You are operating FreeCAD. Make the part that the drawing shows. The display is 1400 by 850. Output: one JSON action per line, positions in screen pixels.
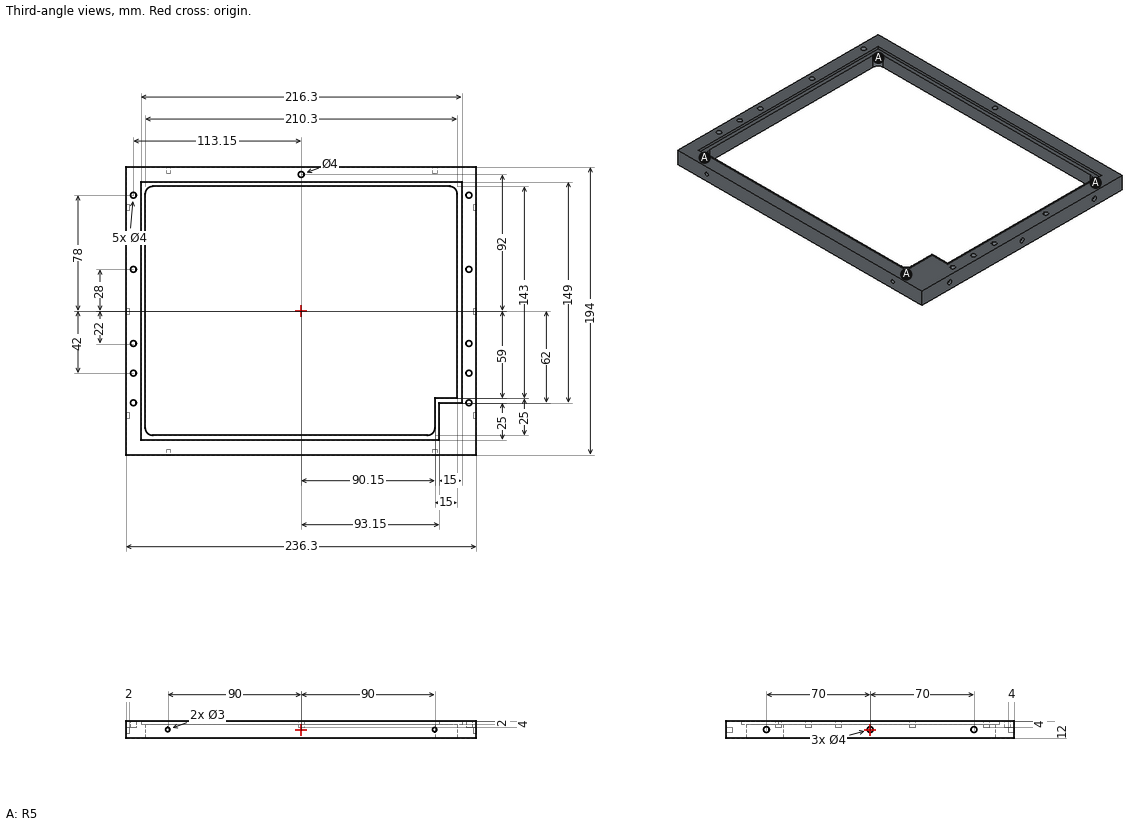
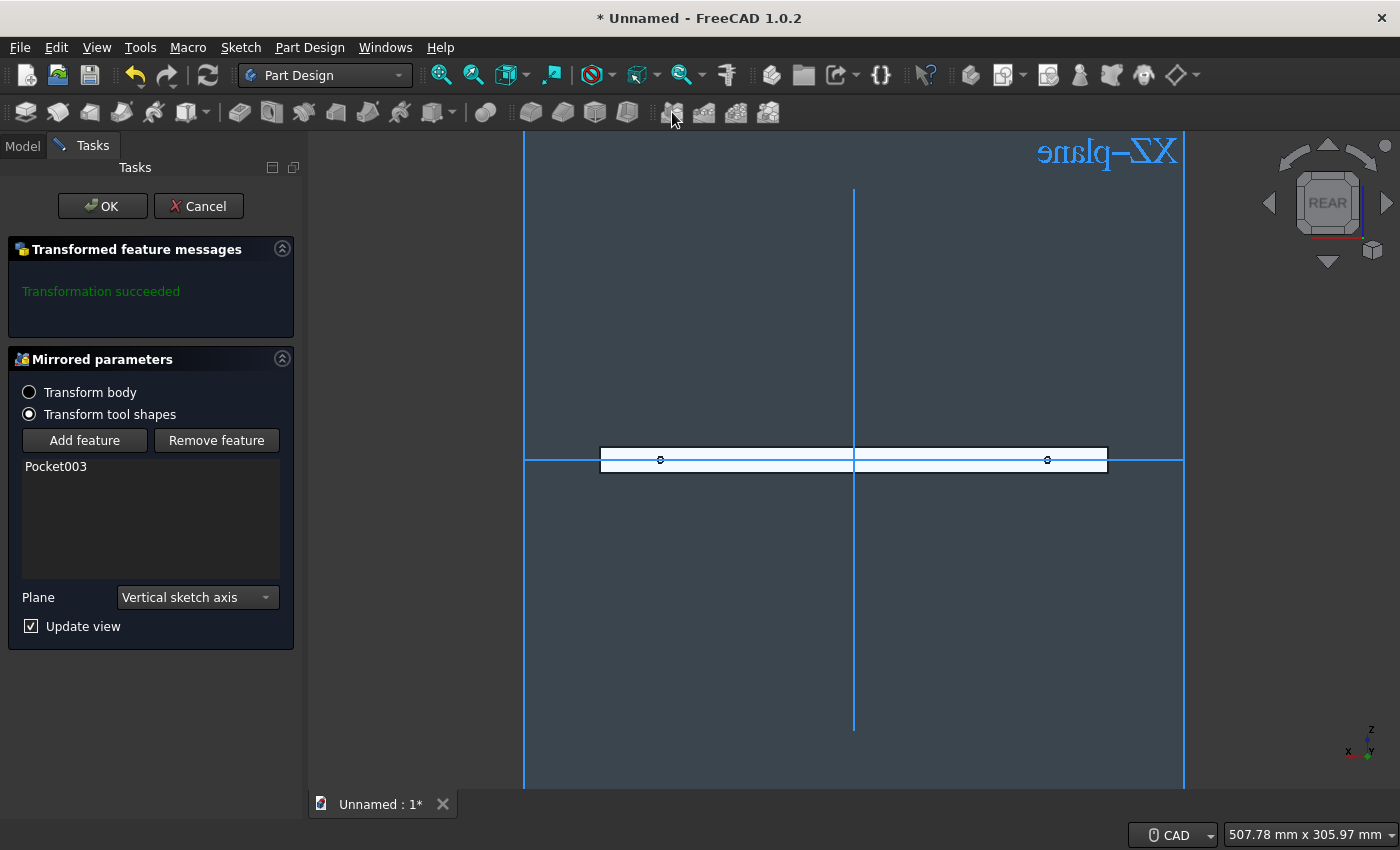
{"action": "left_click", "coordinate": [198, 598]}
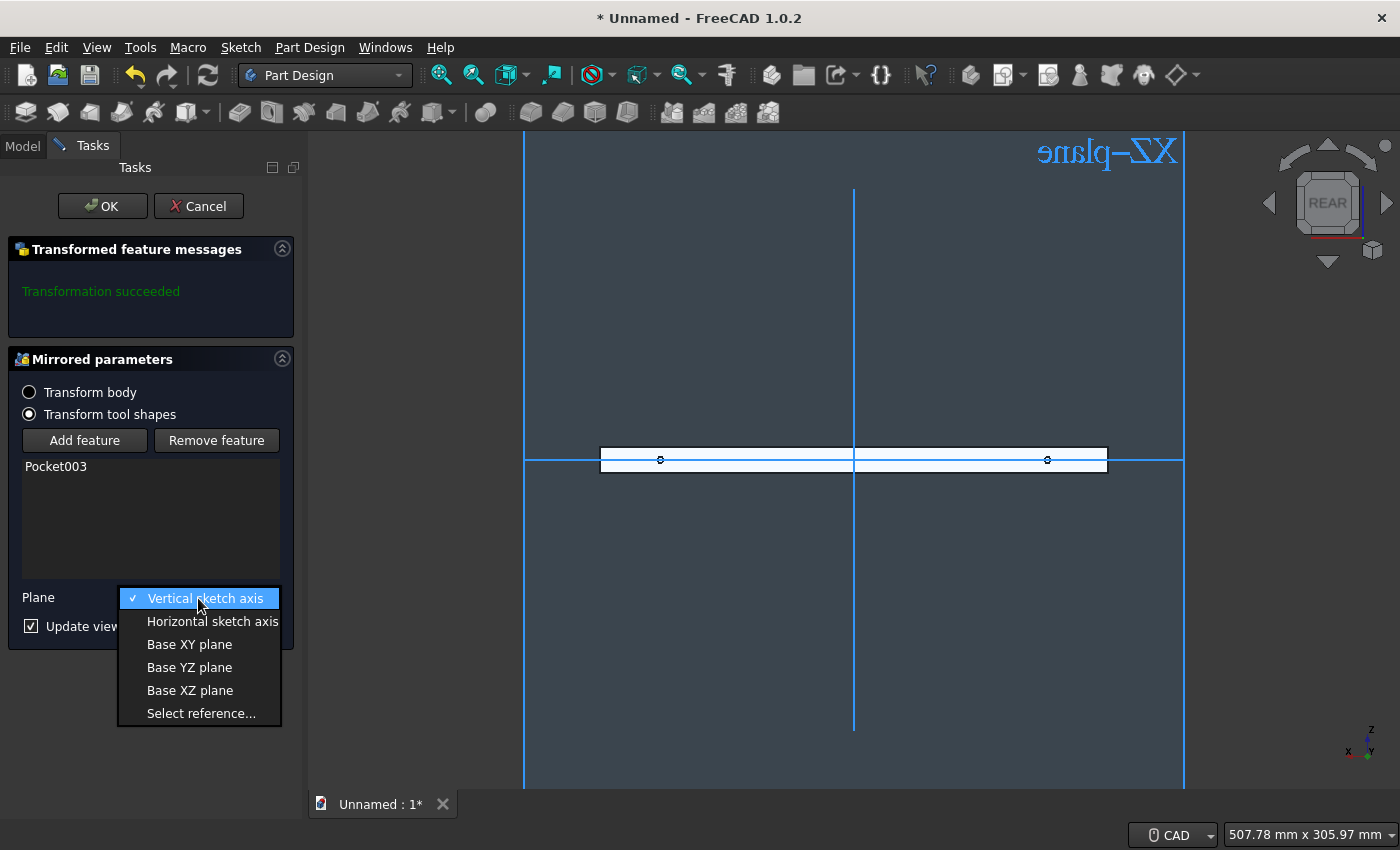
{"action": "left_click", "coordinate": [198, 690]}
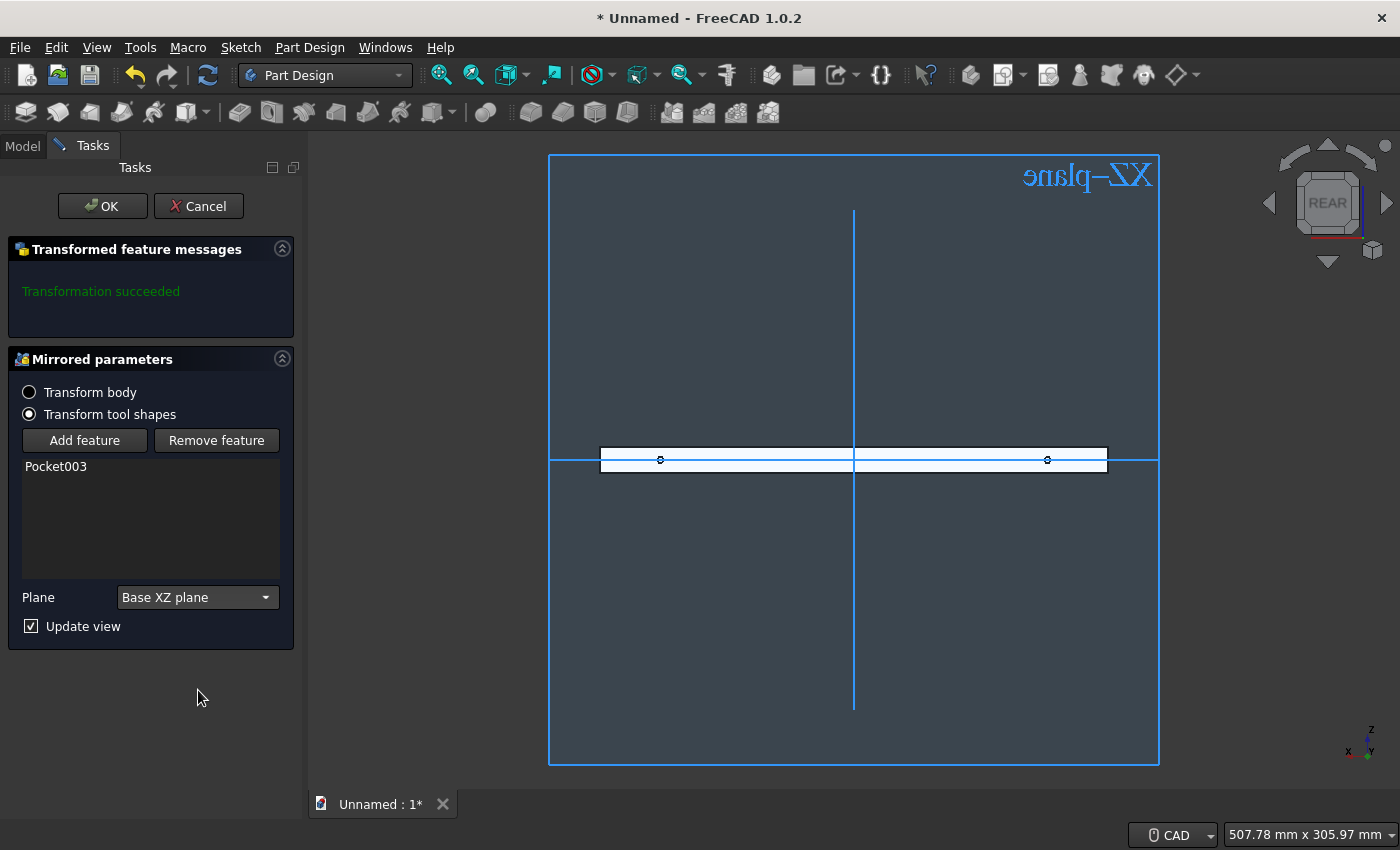
{"action": "left_click", "coordinate": [103, 206]}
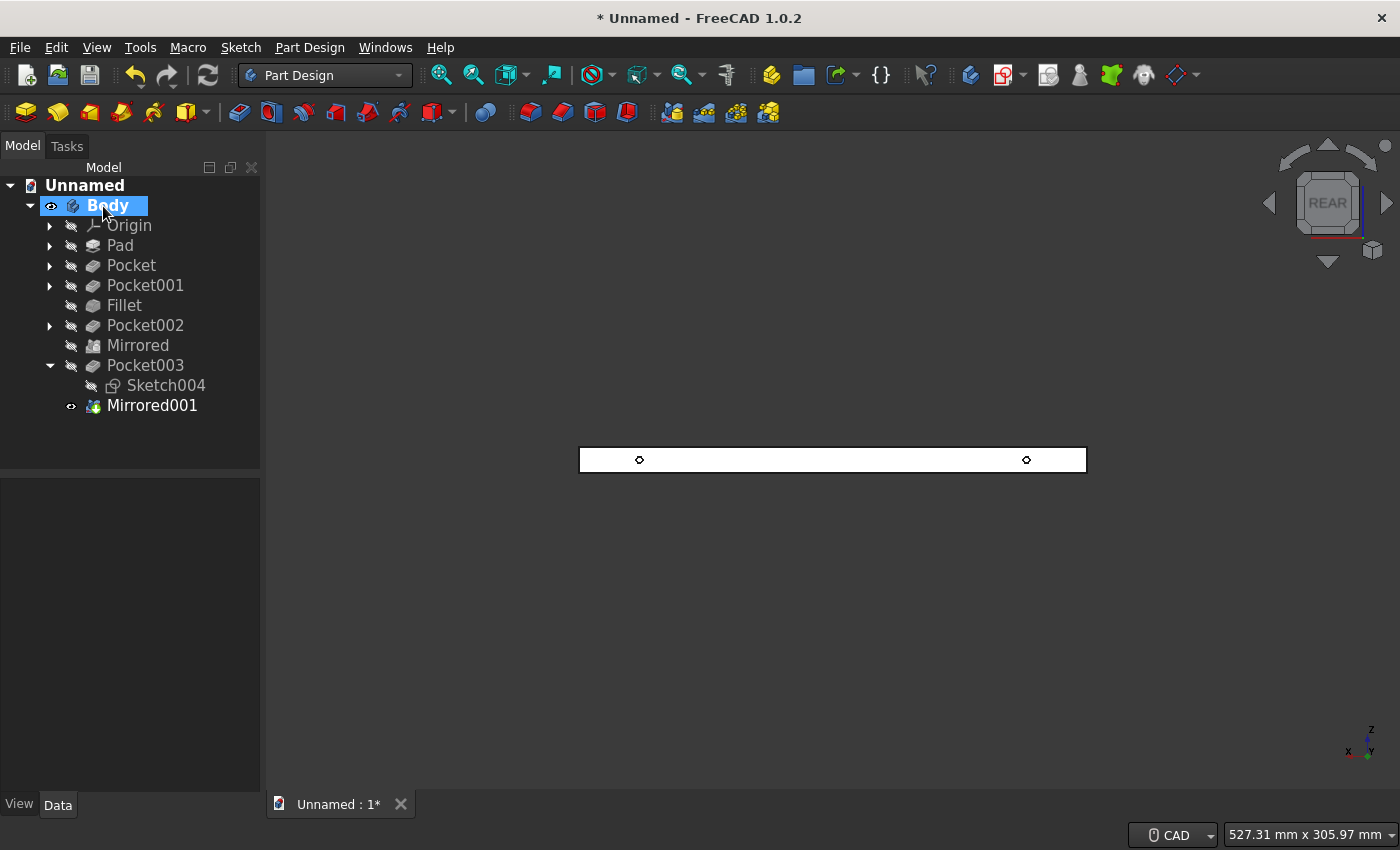
{"action": "left_click", "coordinate": [442, 76]}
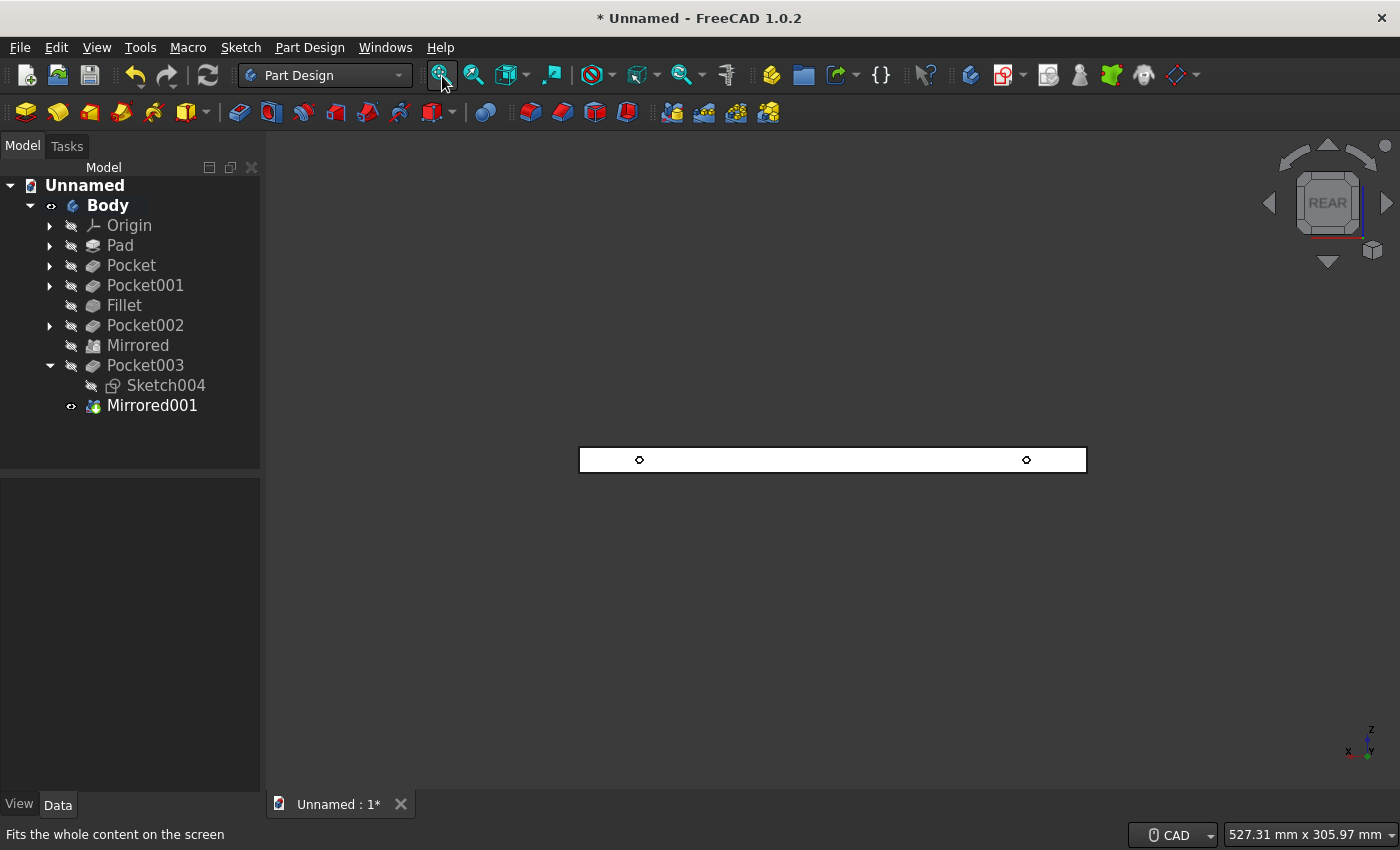
{"action": "key", "text": "0"}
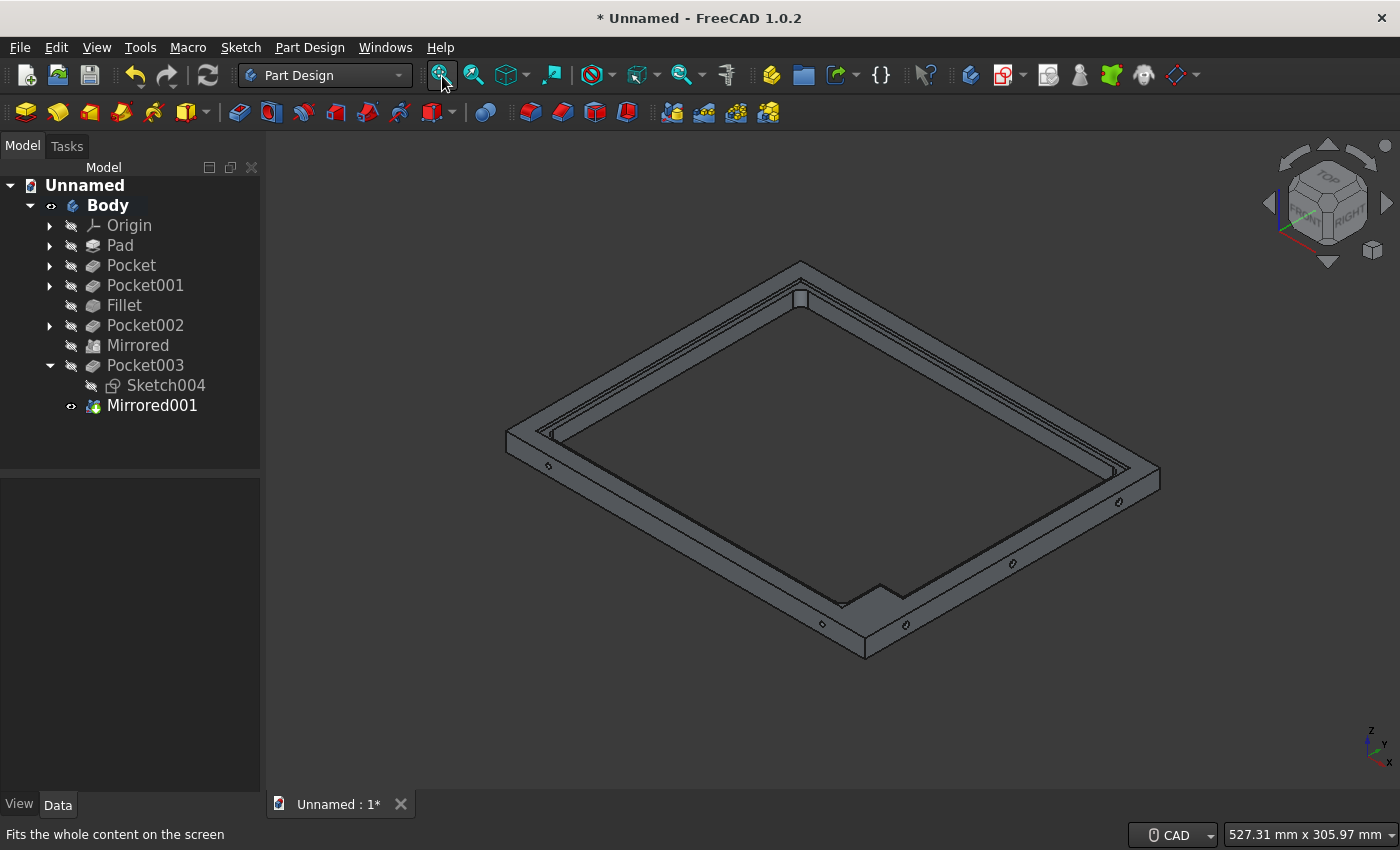
{"action": "left_click", "coordinate": [870, 614]}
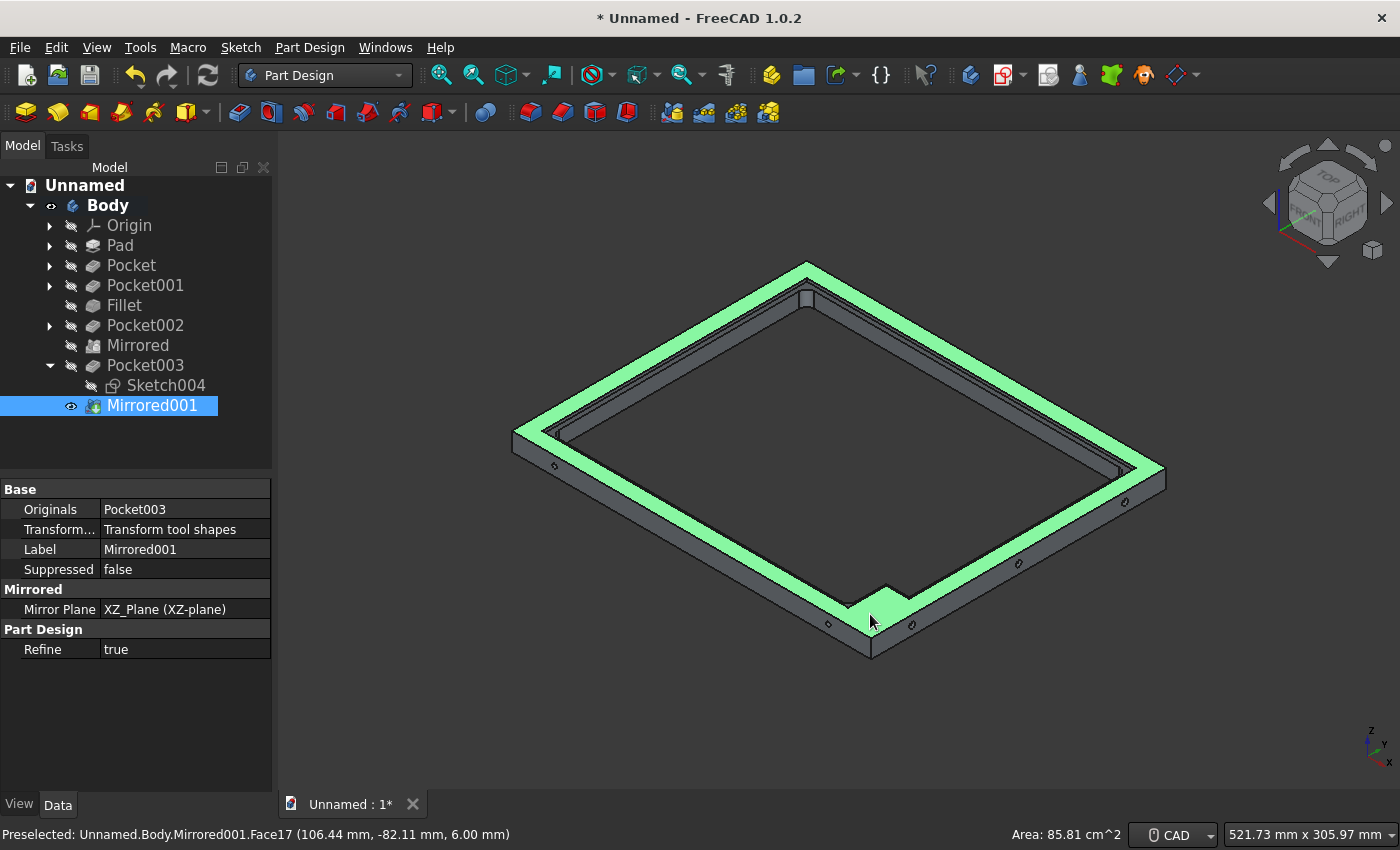
{"action": "left_click", "coordinate": [1004, 76]}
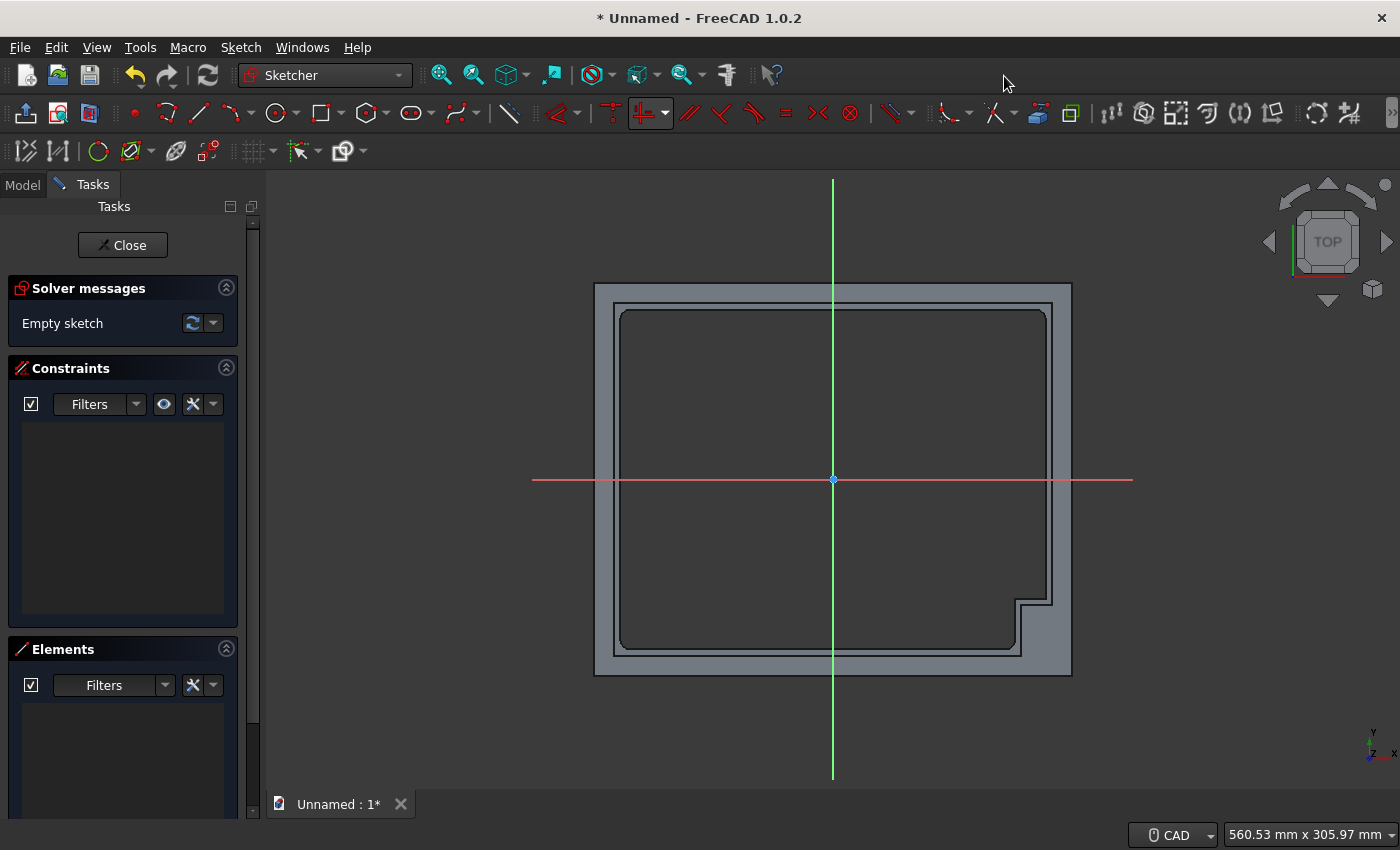
{"action": "scroll", "coordinate": [619, 430], "scroll_direction": "up", "scroll_amount": 2}